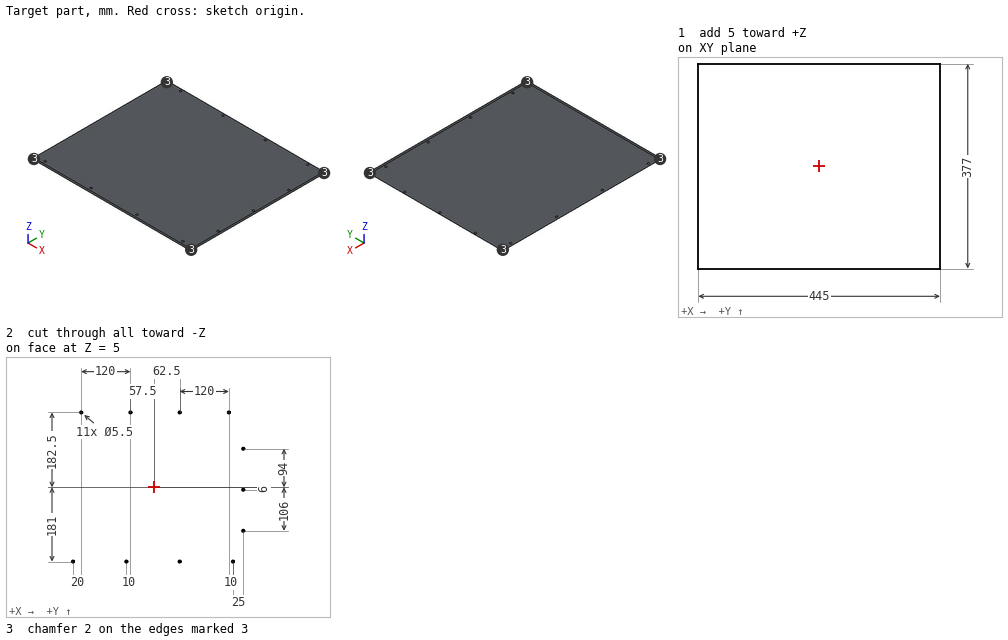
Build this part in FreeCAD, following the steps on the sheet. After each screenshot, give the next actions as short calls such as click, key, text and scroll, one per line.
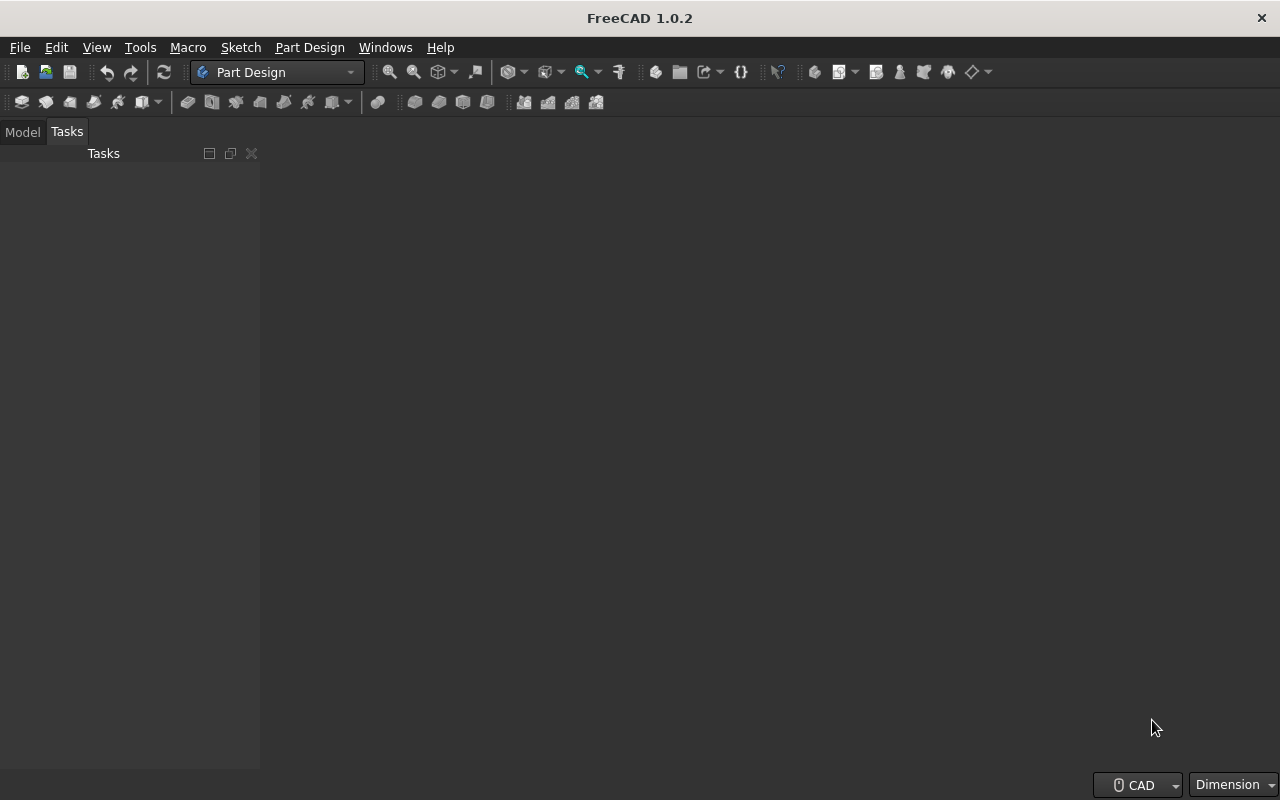
click(22, 72)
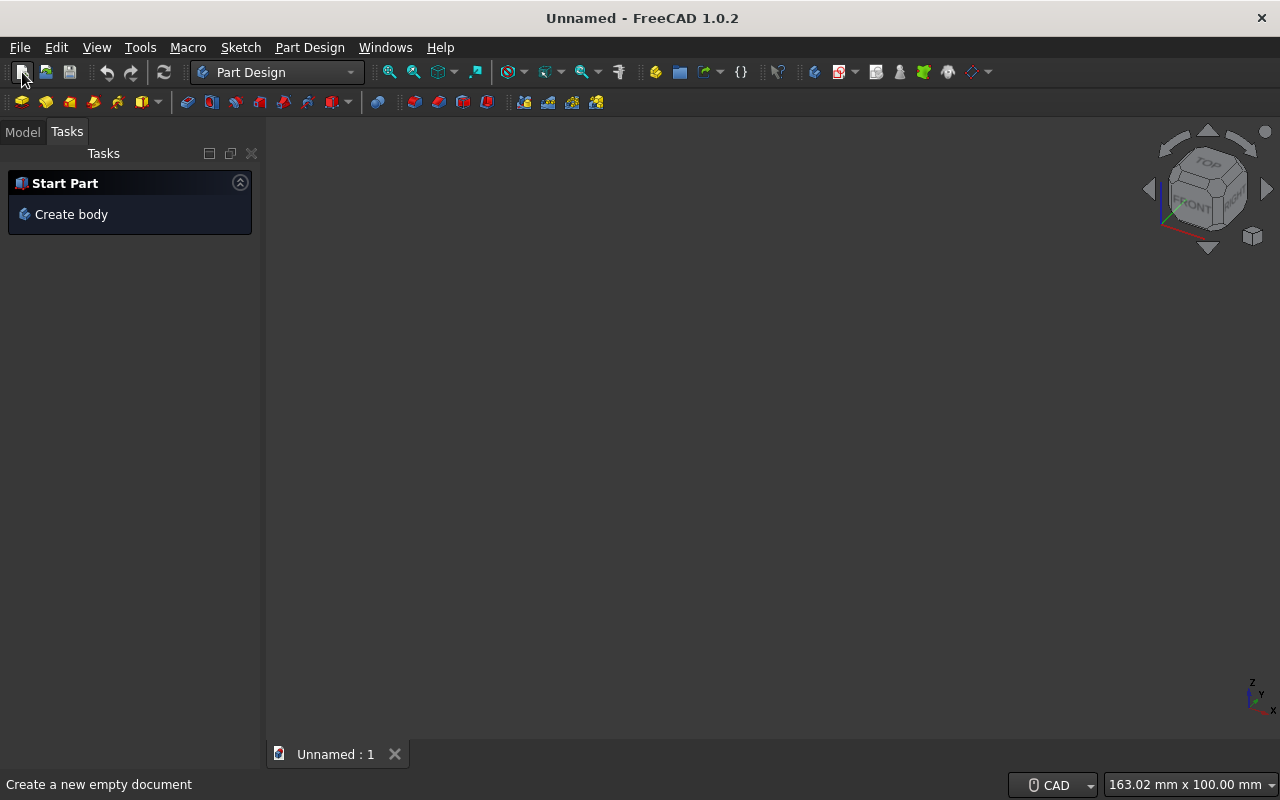
click(840, 72)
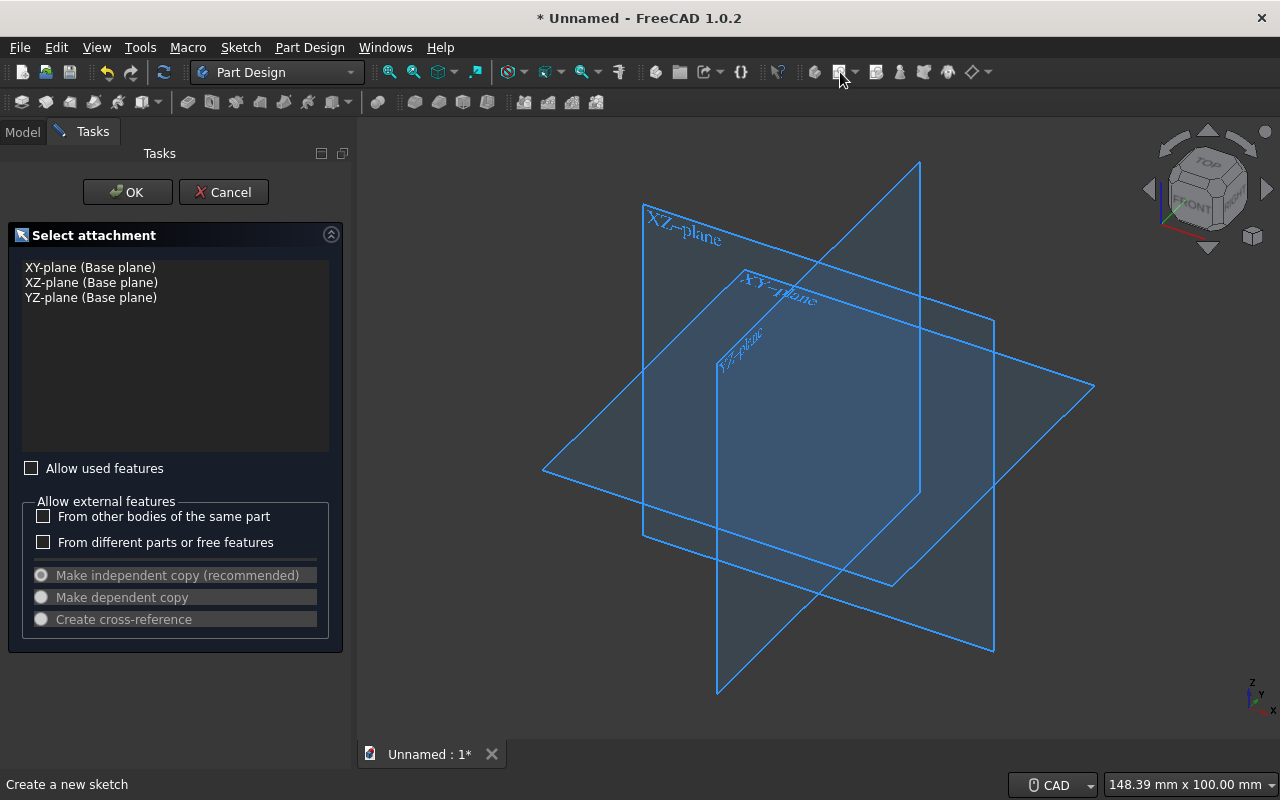
click(82, 268)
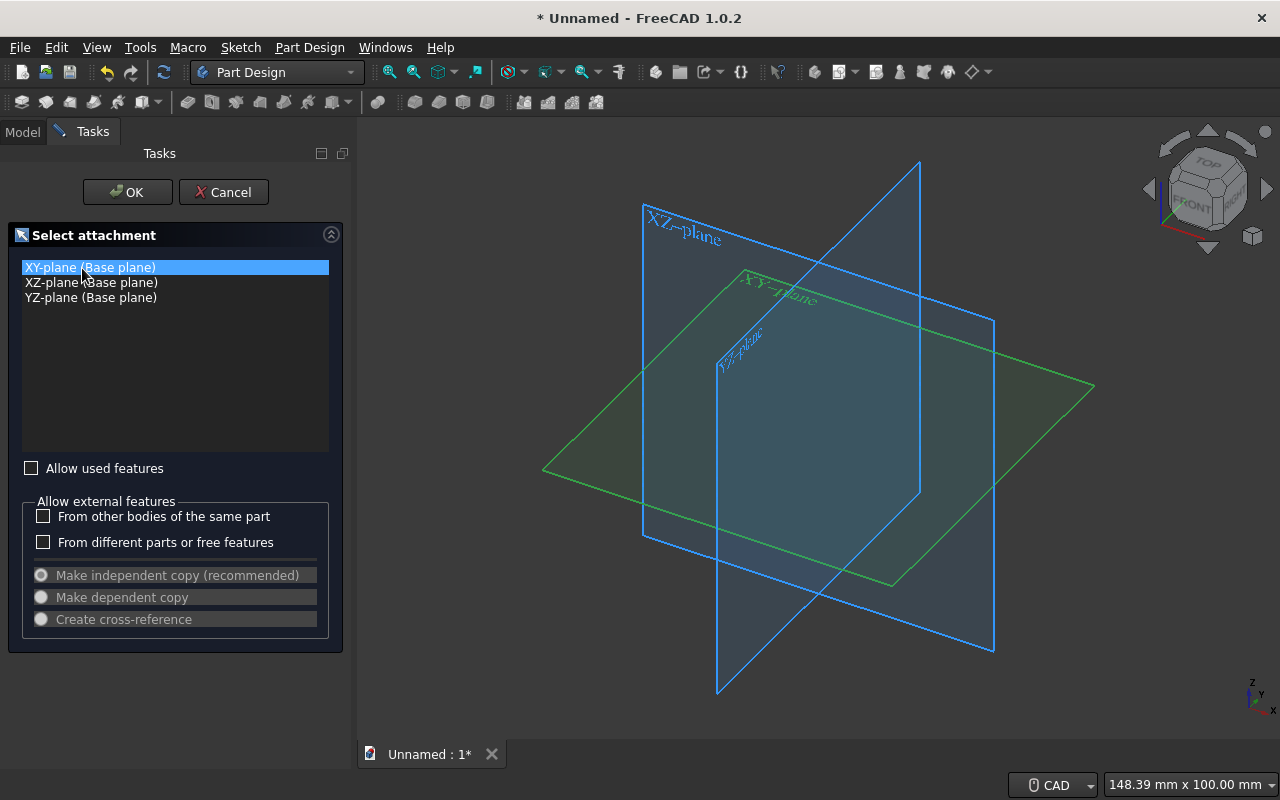
click(128, 192)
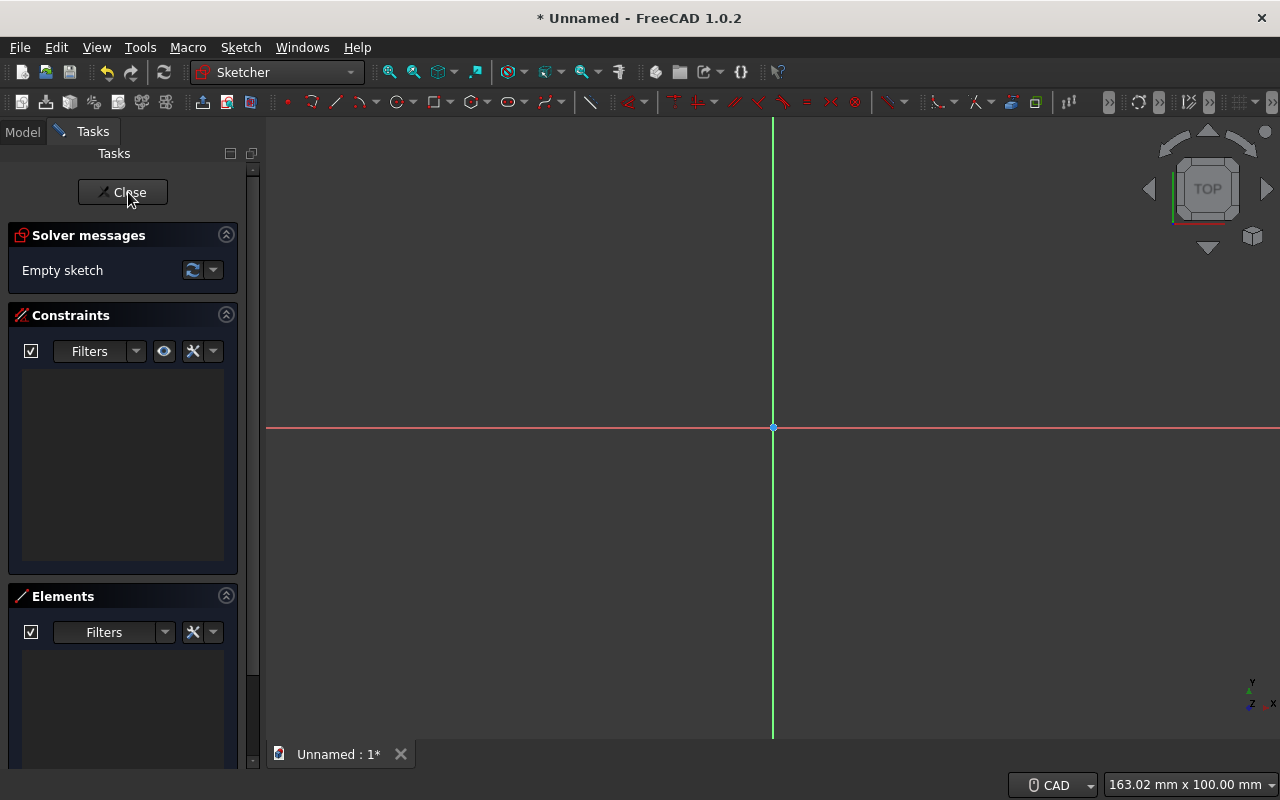
scroll(691, 428, down, 9)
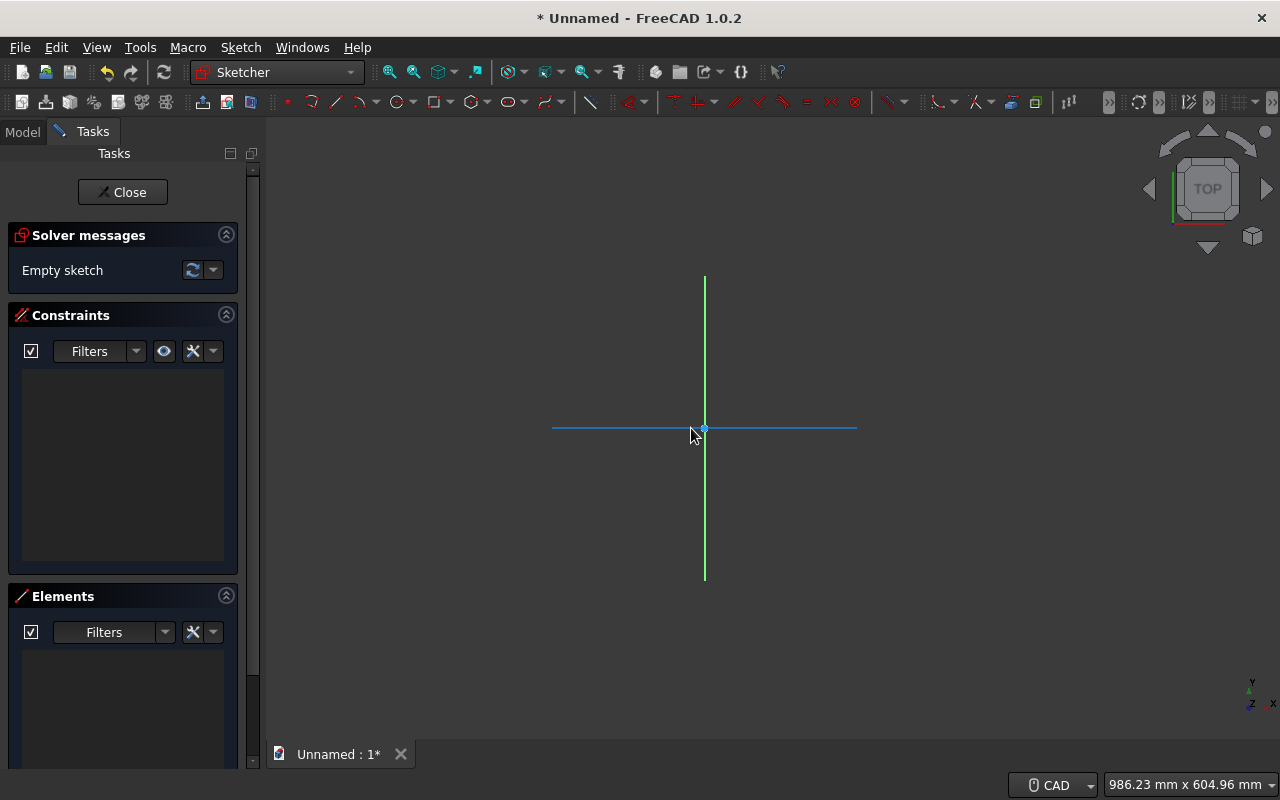
key(g)
key(v)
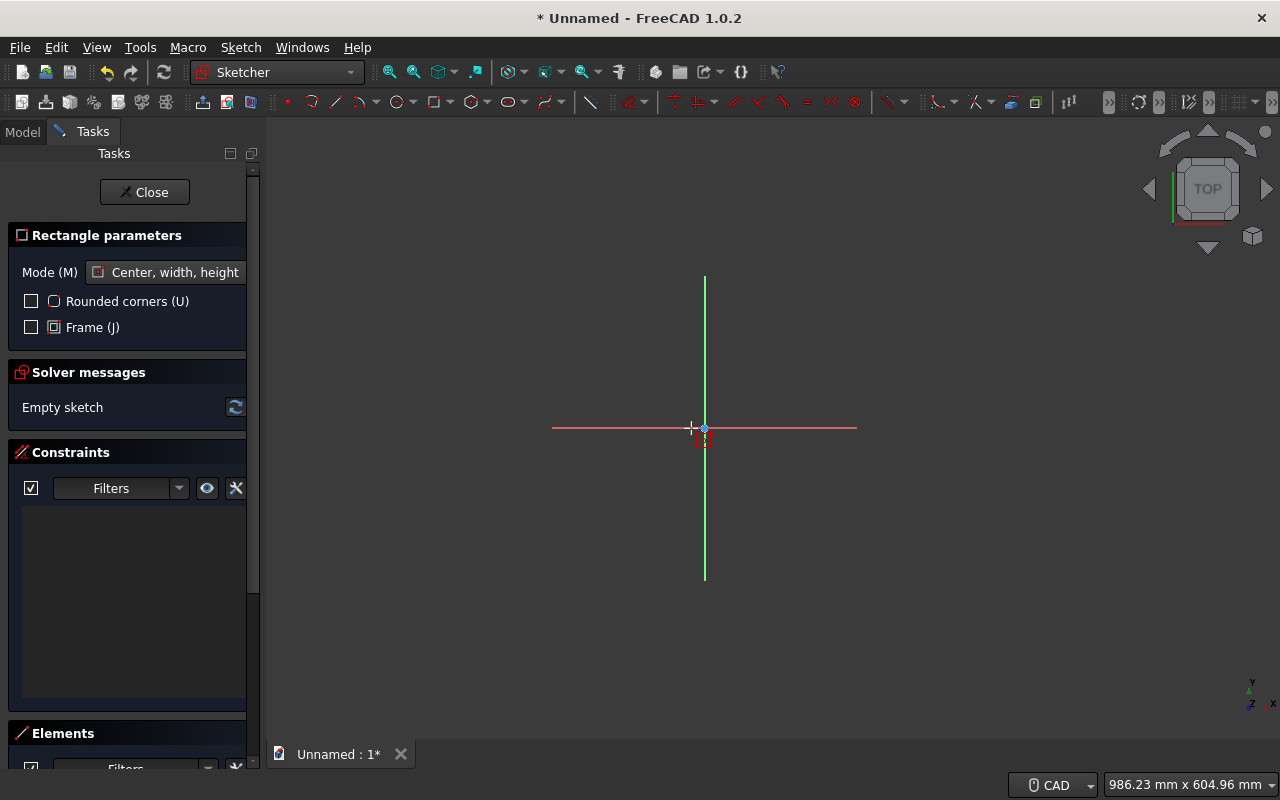
click(705, 428)
move(934, 235)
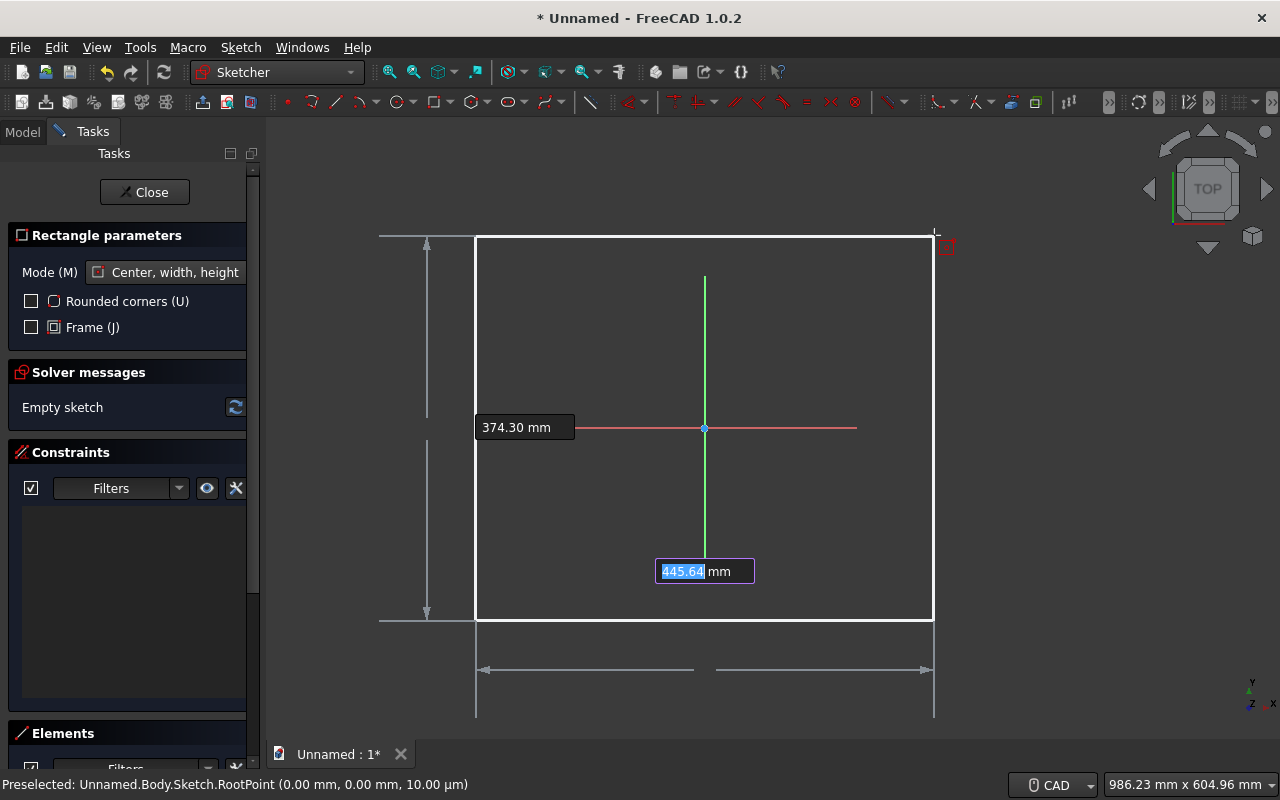
text(445)
key(Tab)
text(377)
key(Return)
key(Escape)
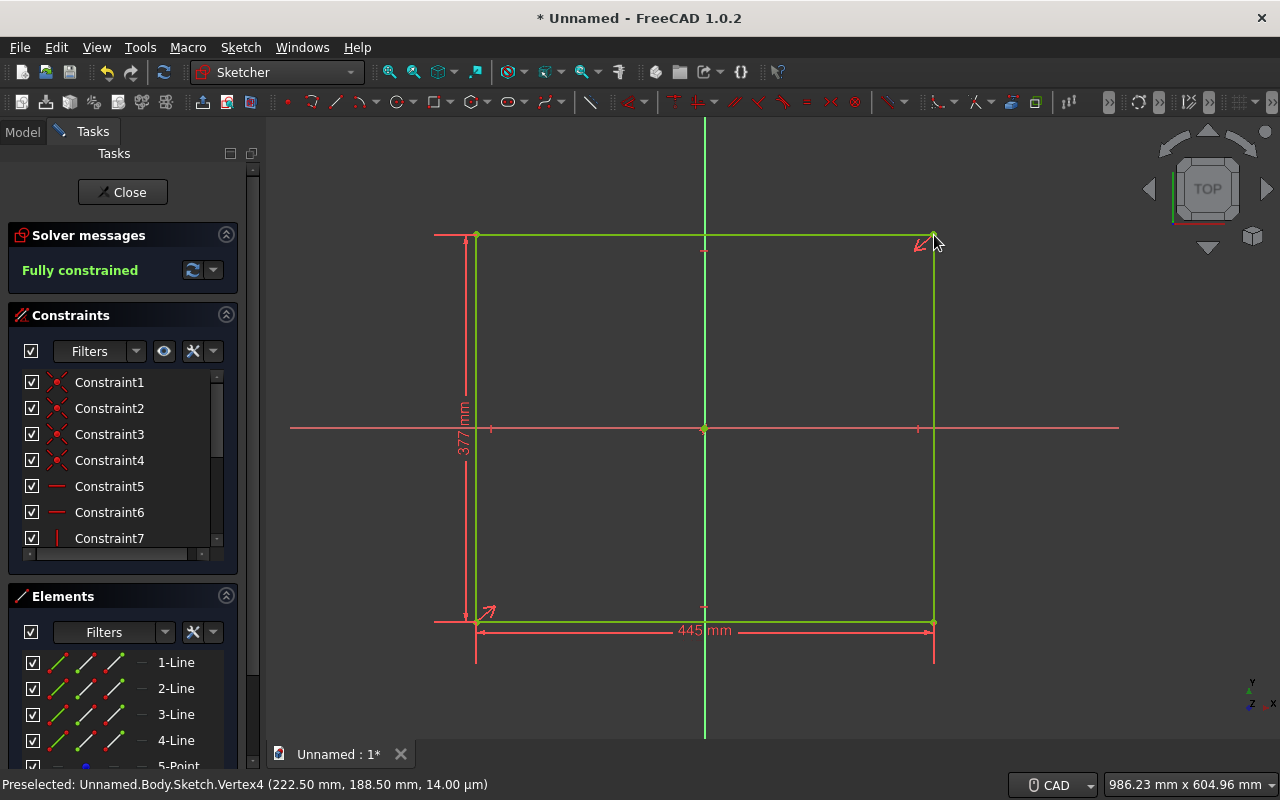
click(123, 192)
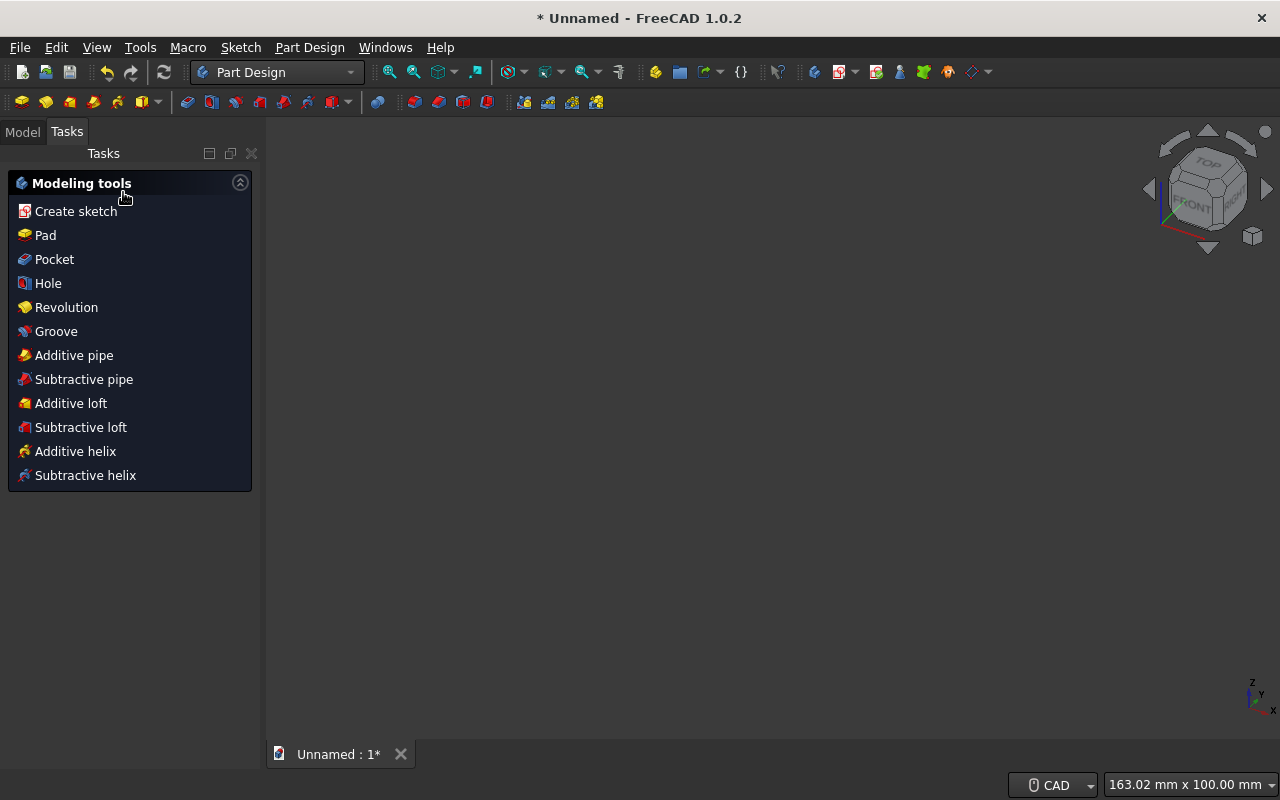
click(22, 102)